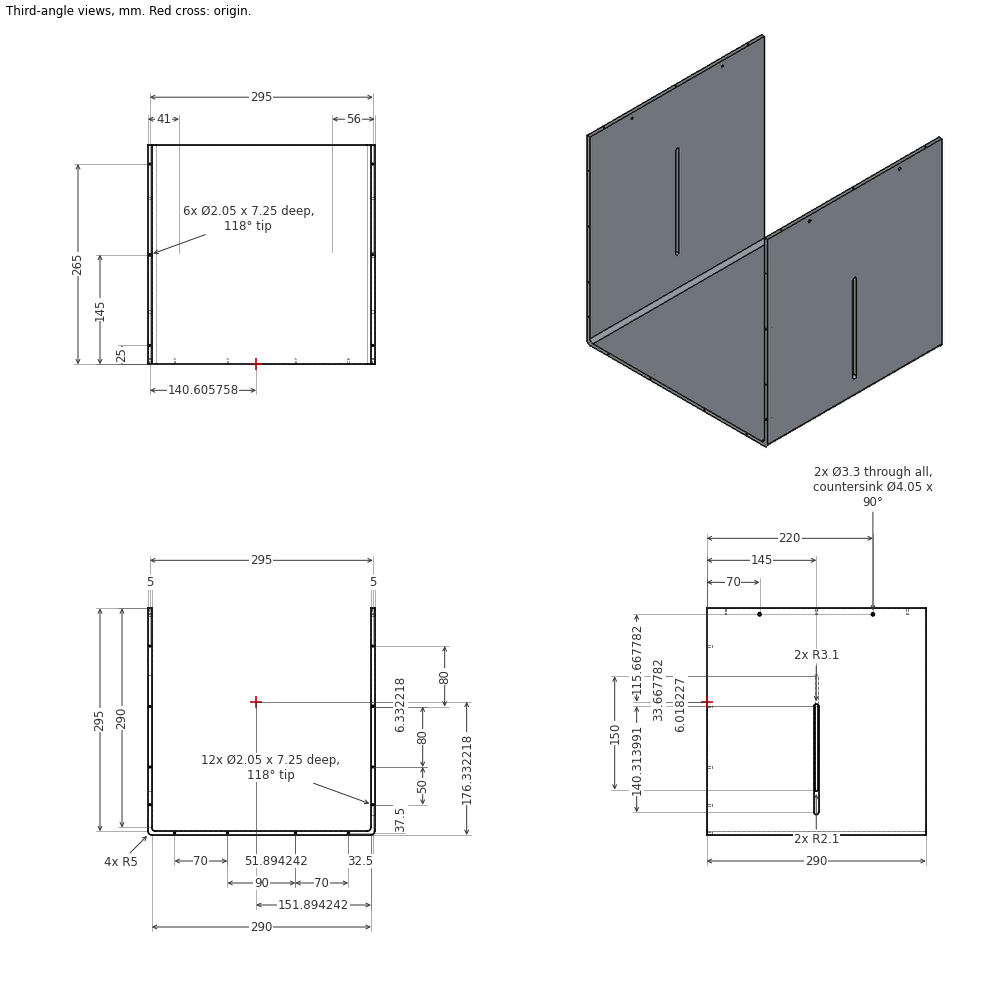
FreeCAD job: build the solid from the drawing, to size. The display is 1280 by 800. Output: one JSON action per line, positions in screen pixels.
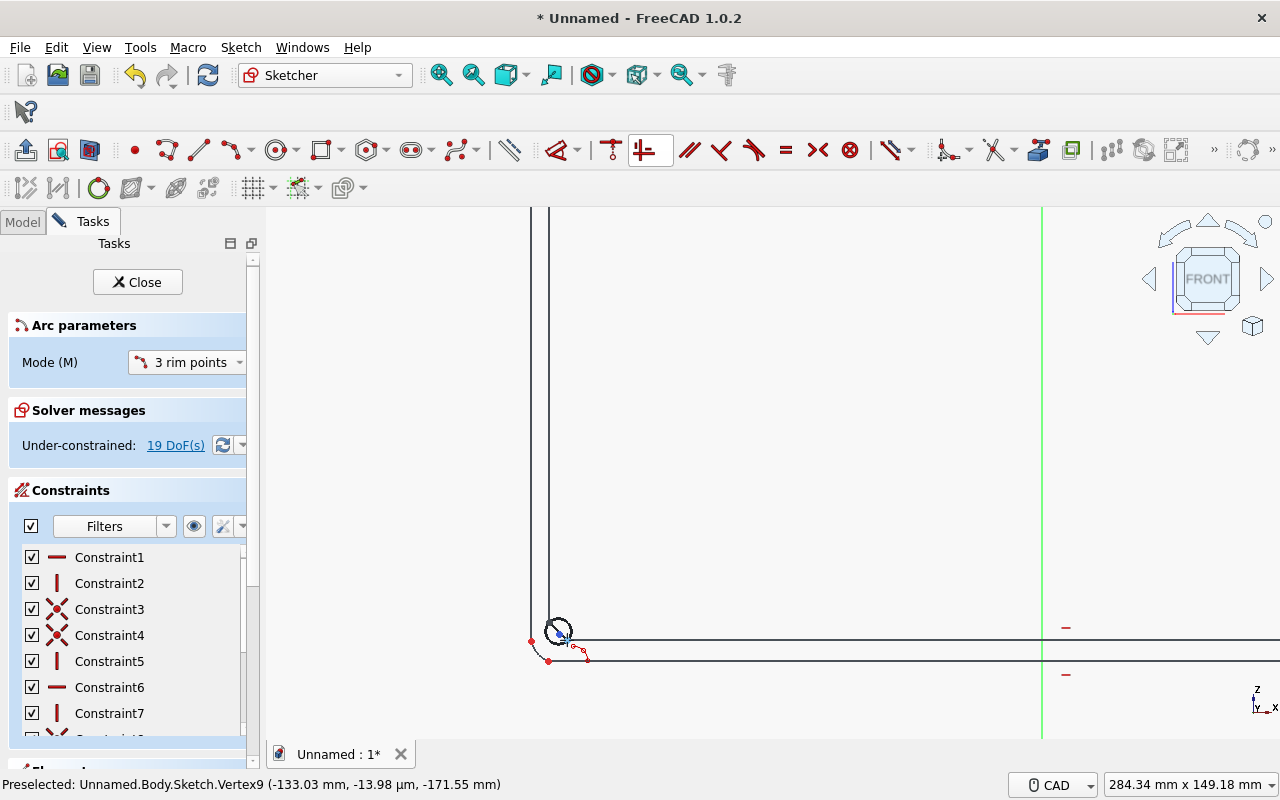
{"action": "scroll", "coordinate": [555, 634], "scroll_direction": "up", "scroll_amount": 6}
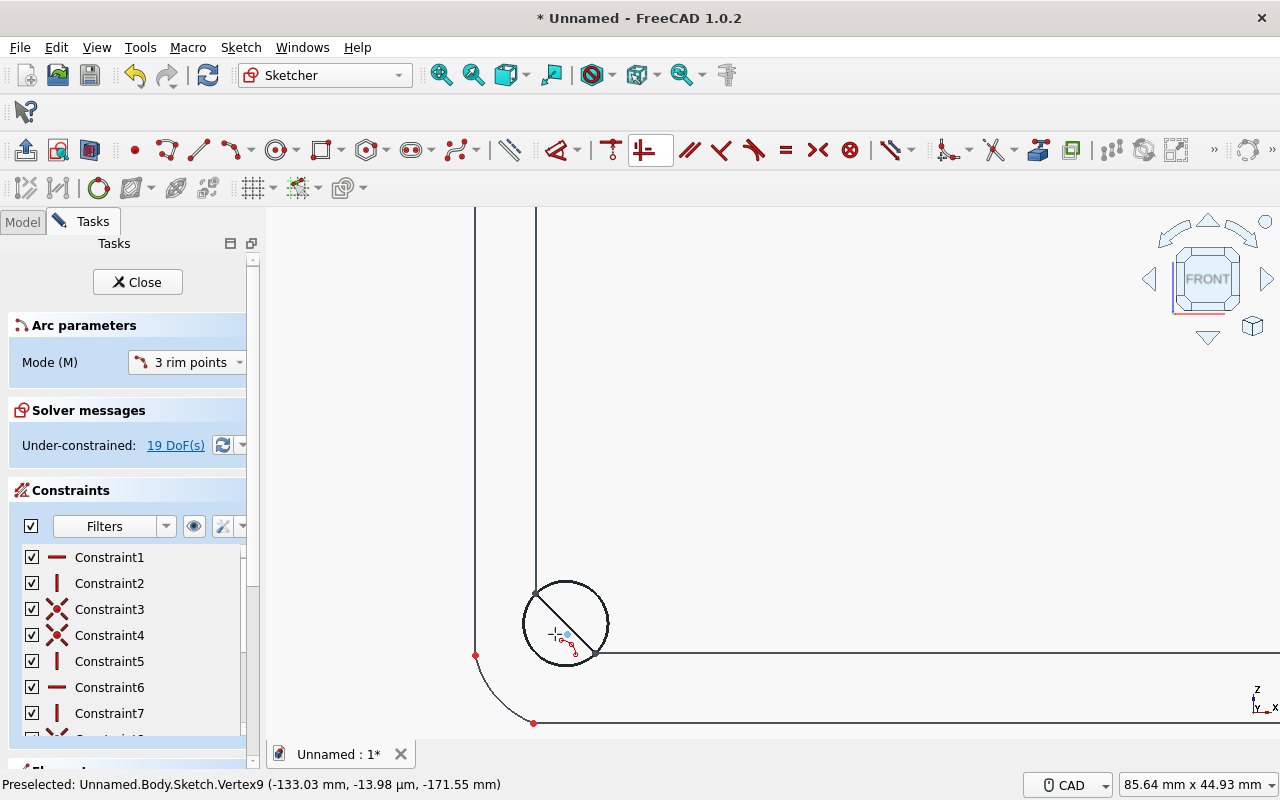
{"action": "left_click", "coordinate": [553, 634]}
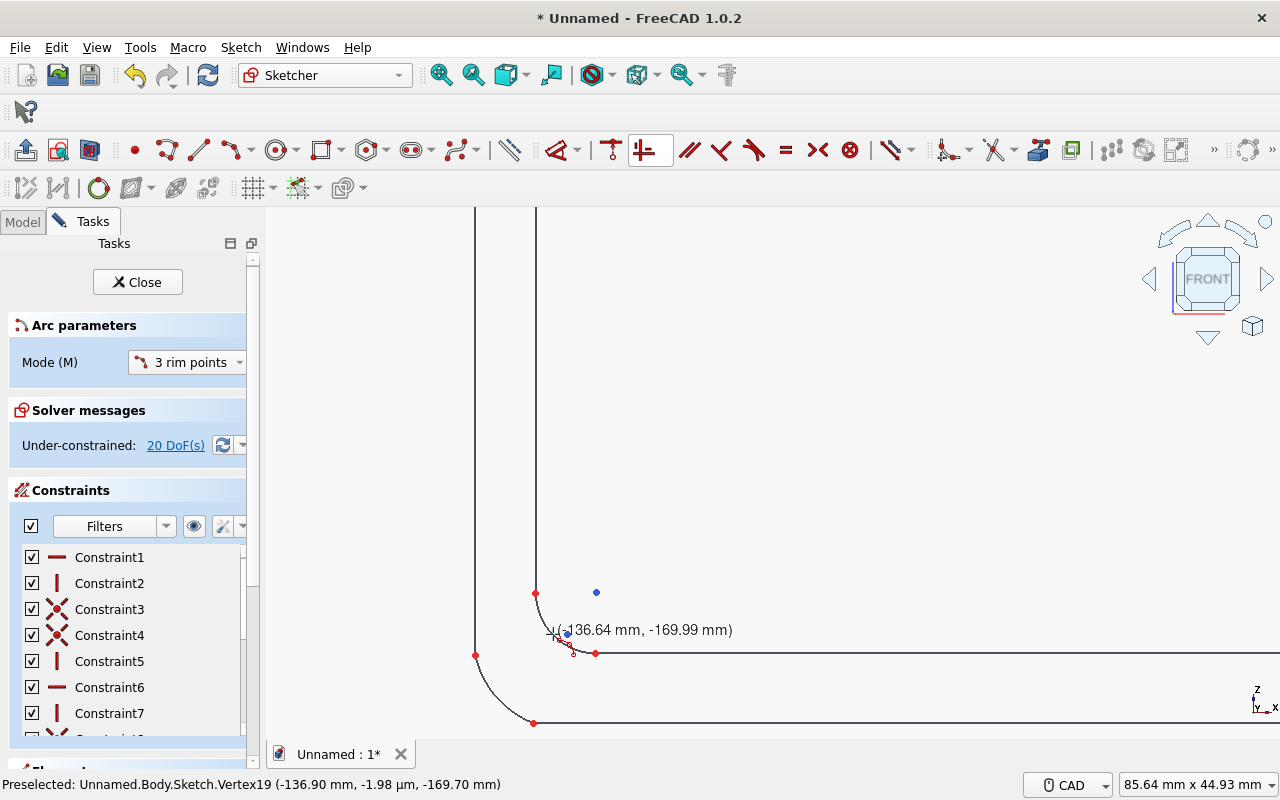
{"action": "scroll", "coordinate": [550, 627], "scroll_direction": "down", "scroll_amount": 12}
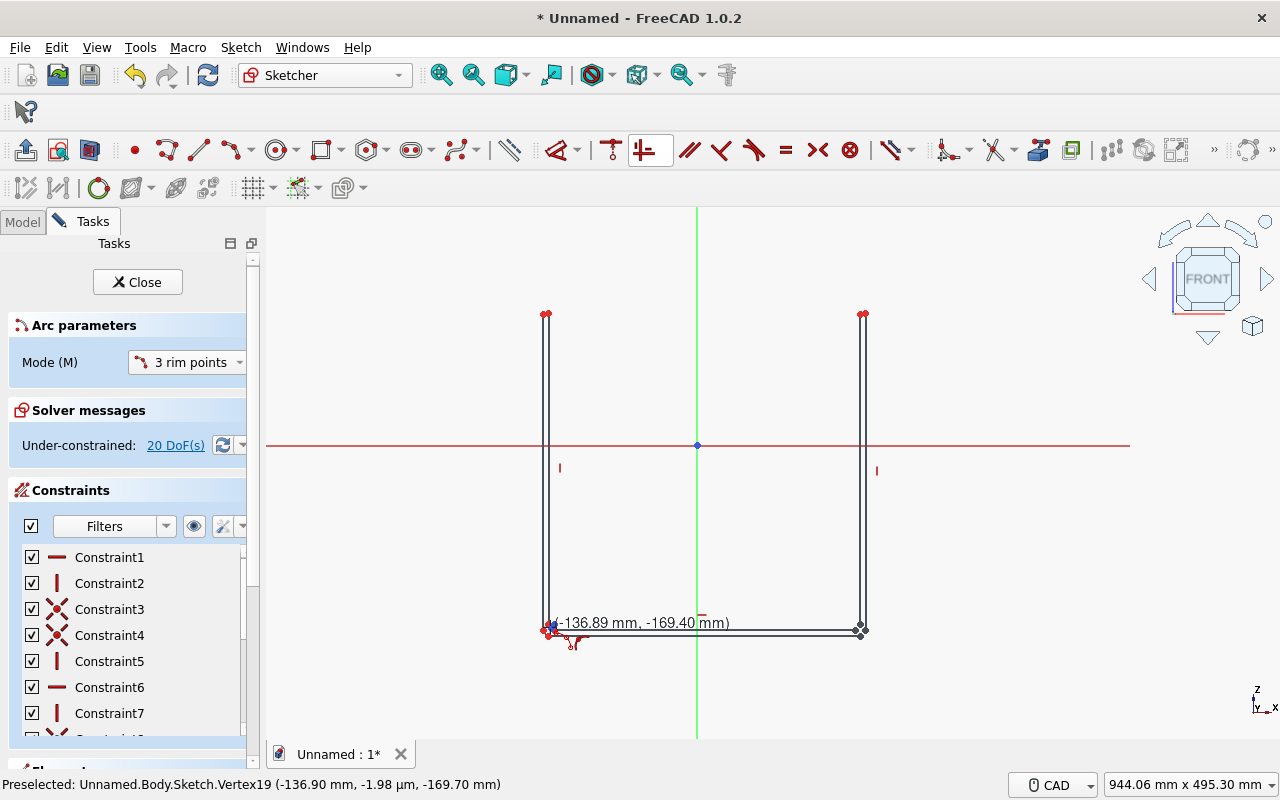
{"action": "scroll", "coordinate": [855, 630], "scroll_direction": "up", "scroll_amount": 6}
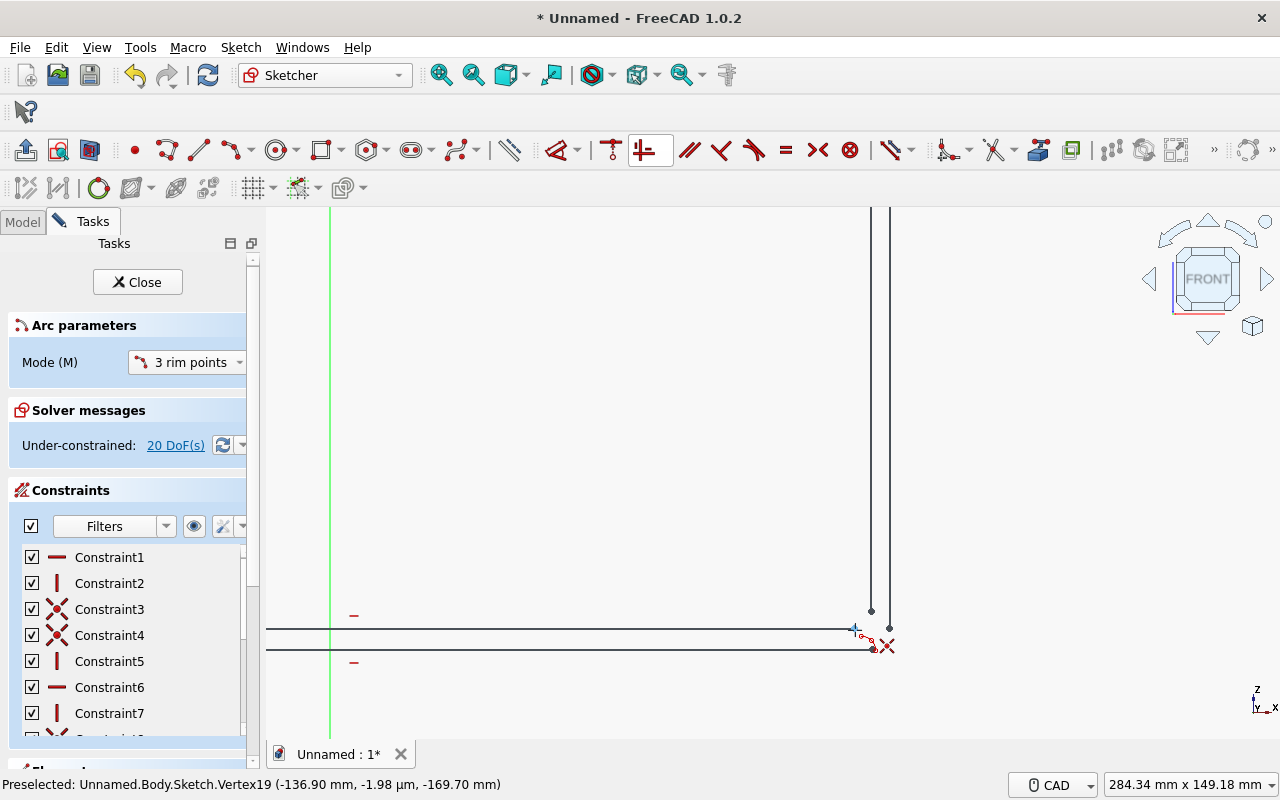
{"action": "left_click", "coordinate": [854, 629]}
{"action": "left_click", "coordinate": [871, 611]}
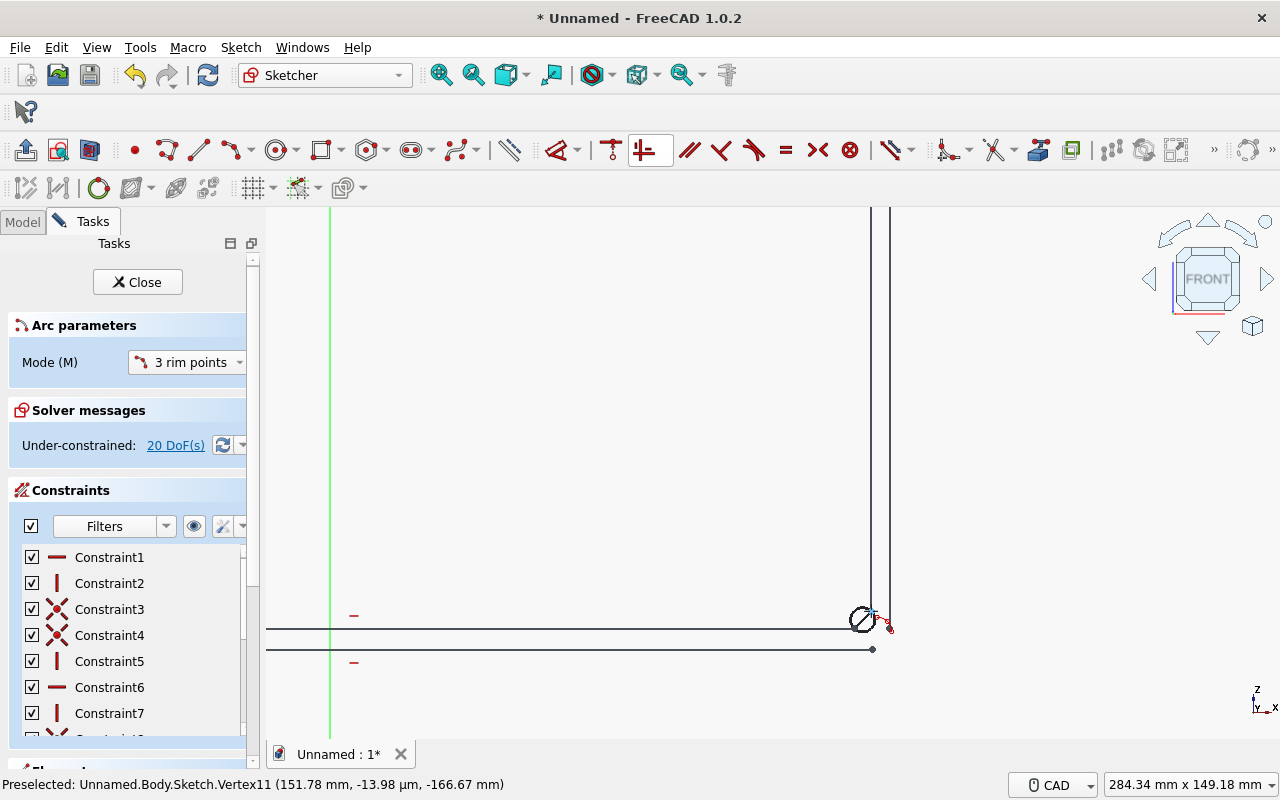
{"action": "scroll", "coordinate": [866, 623], "scroll_direction": "up", "scroll_amount": 6}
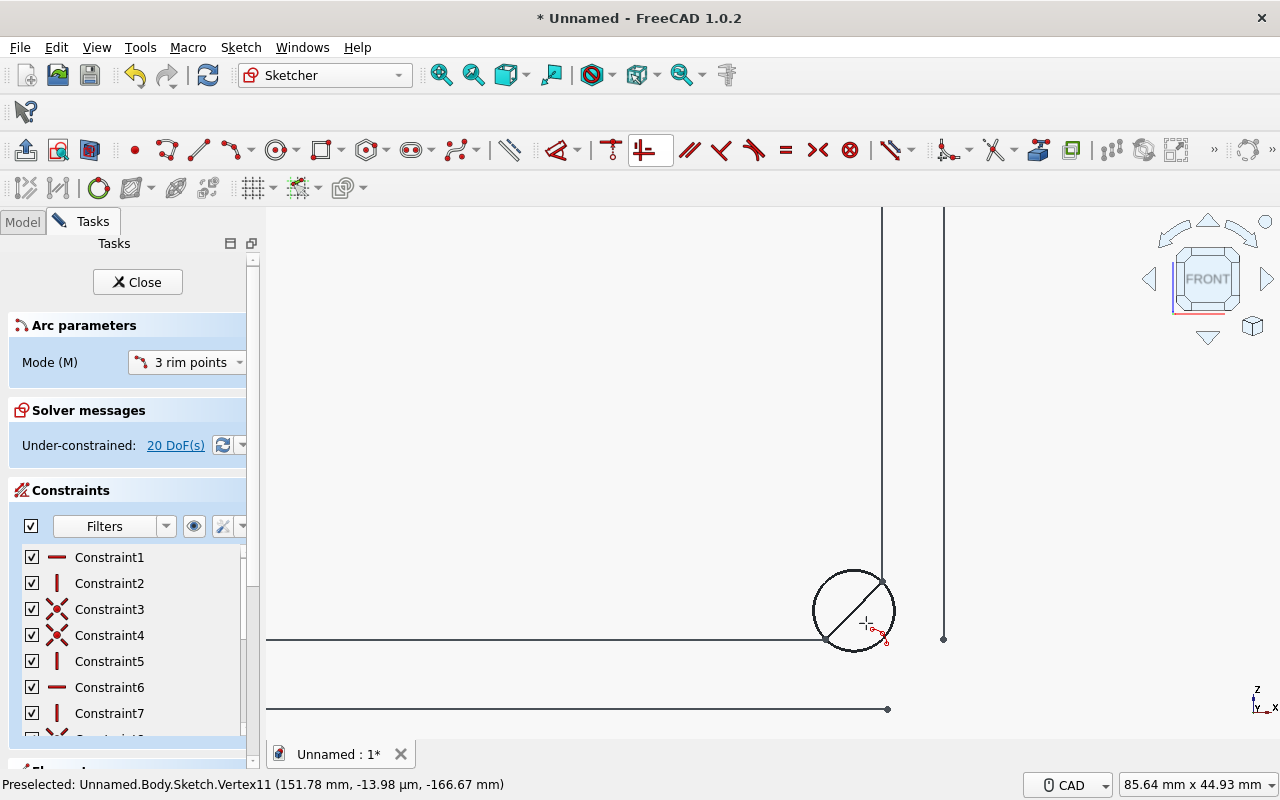
{"action": "left_click", "coordinate": [866, 620]}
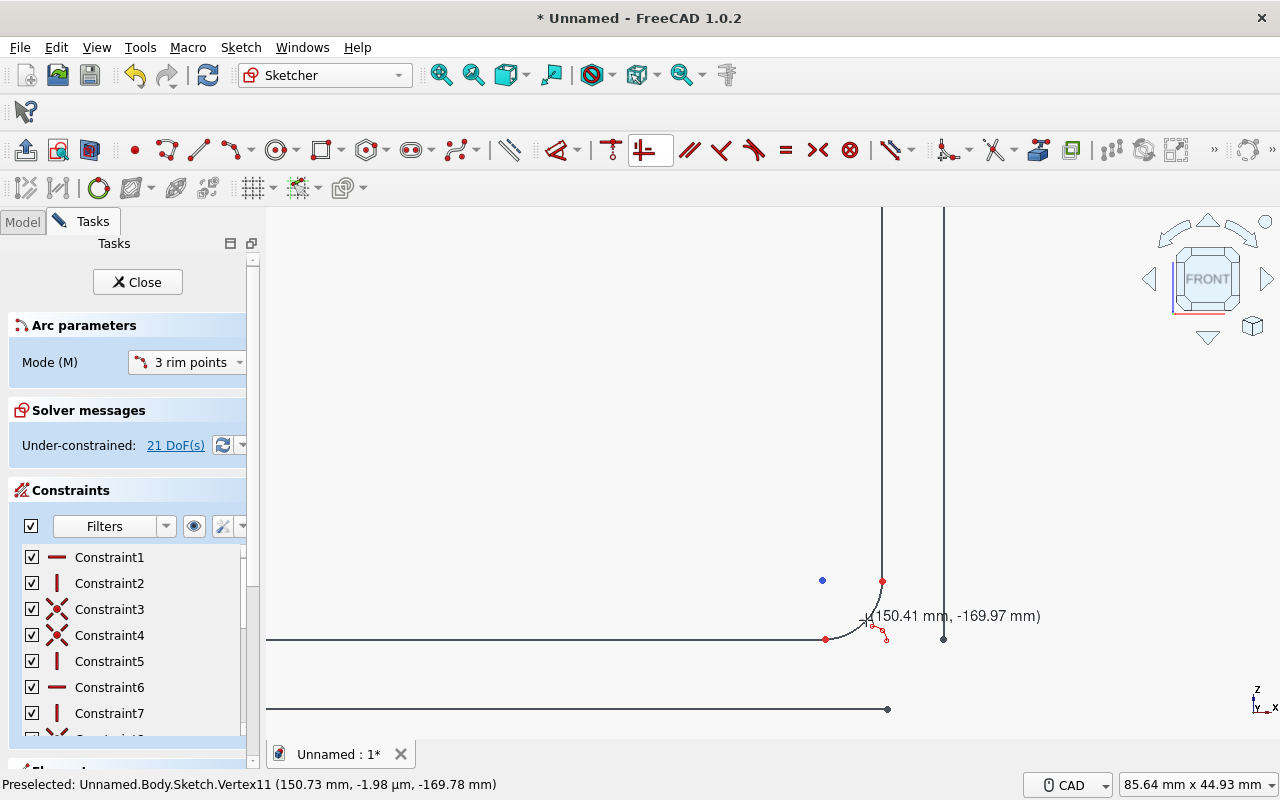
{"action": "scroll", "coordinate": [858, 628], "scroll_direction": "down", "scroll_amount": 12}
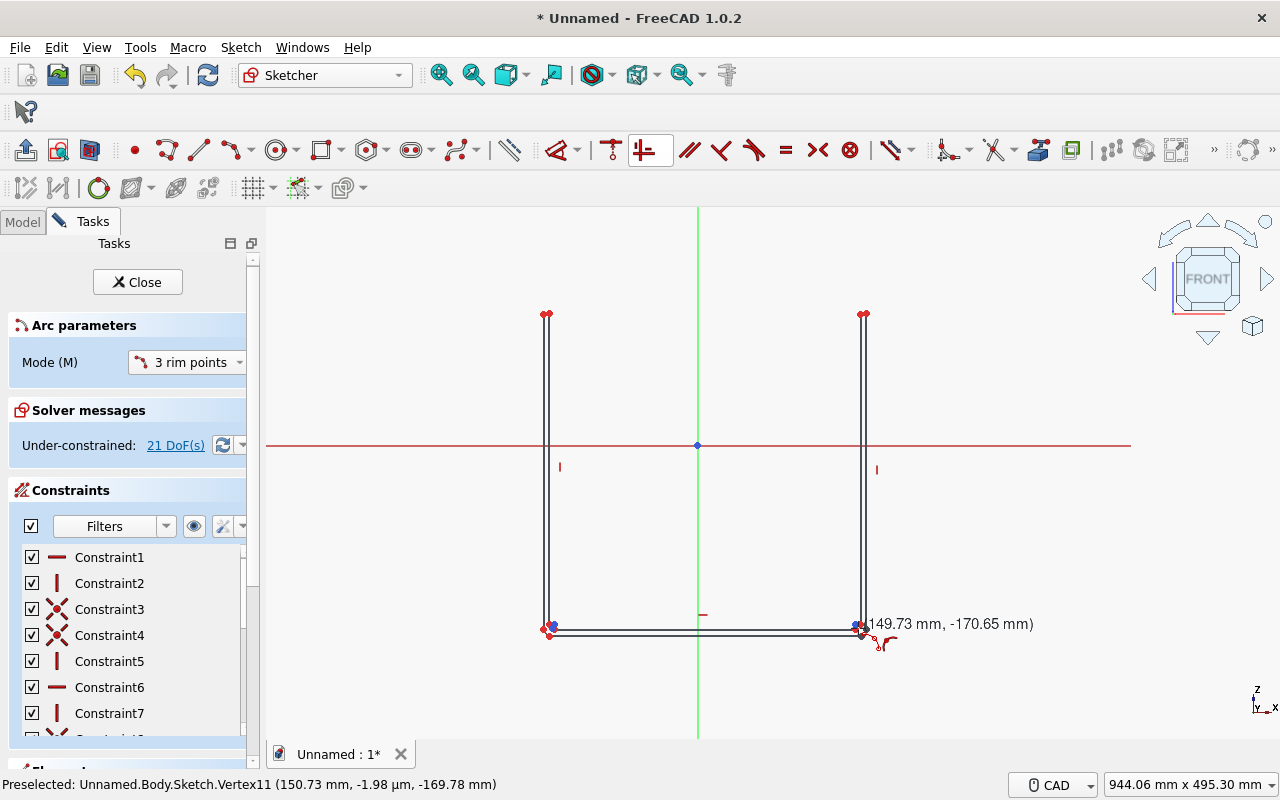
{"action": "scroll", "coordinate": [866, 630], "scroll_direction": "up", "scroll_amount": 5}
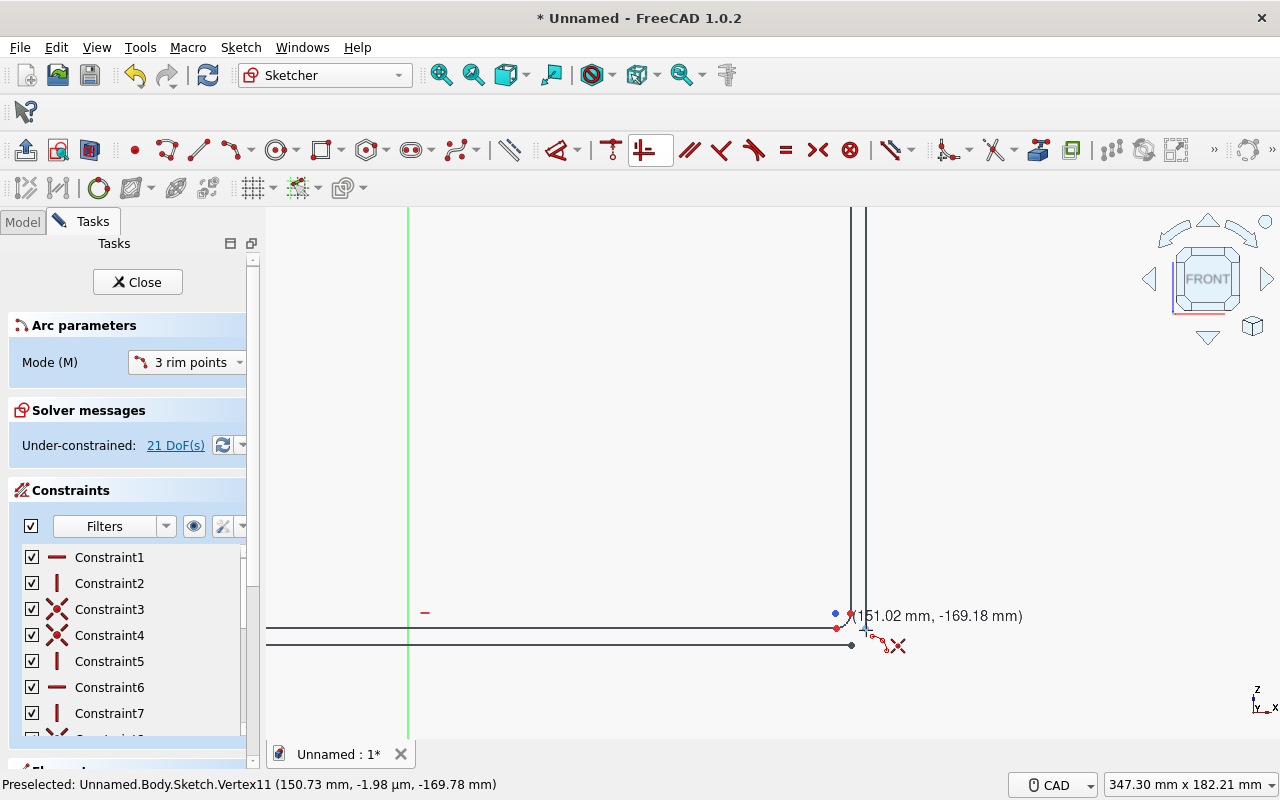
{"action": "left_click", "coordinate": [866, 628]}
{"action": "left_click", "coordinate": [852, 645]}